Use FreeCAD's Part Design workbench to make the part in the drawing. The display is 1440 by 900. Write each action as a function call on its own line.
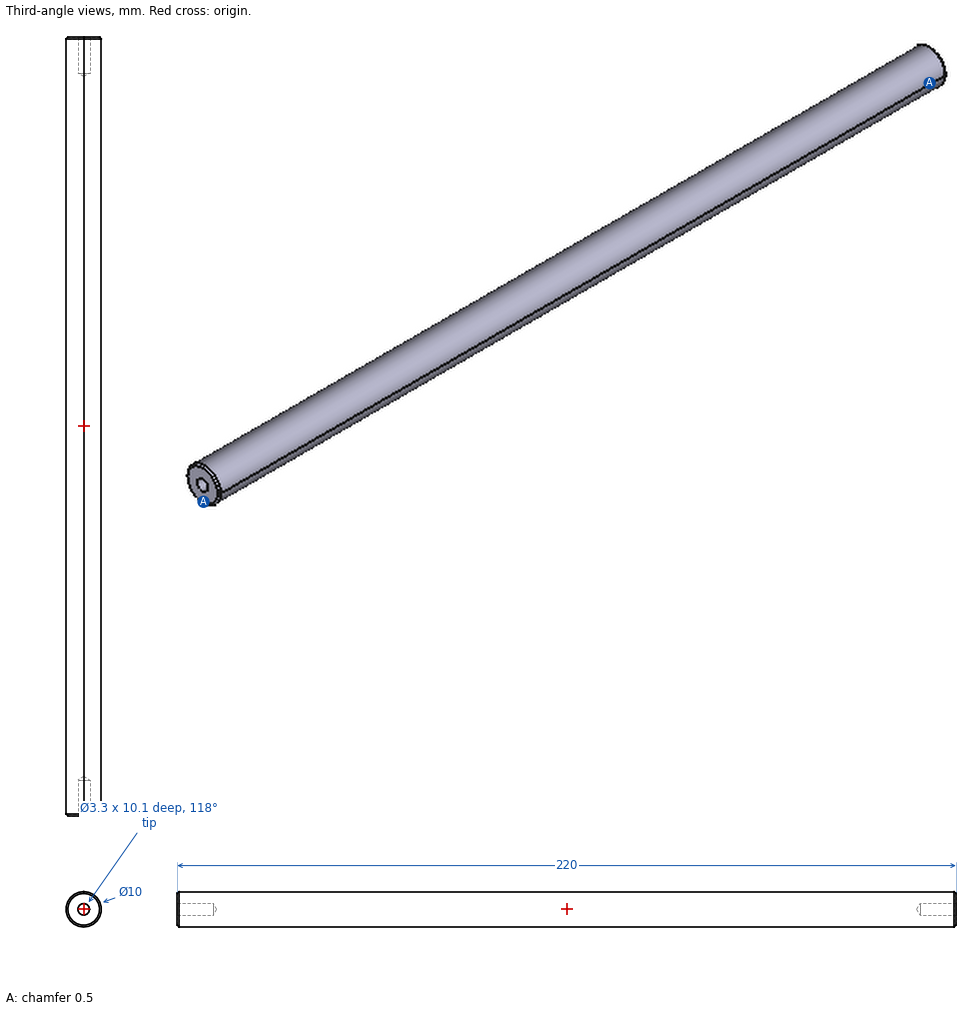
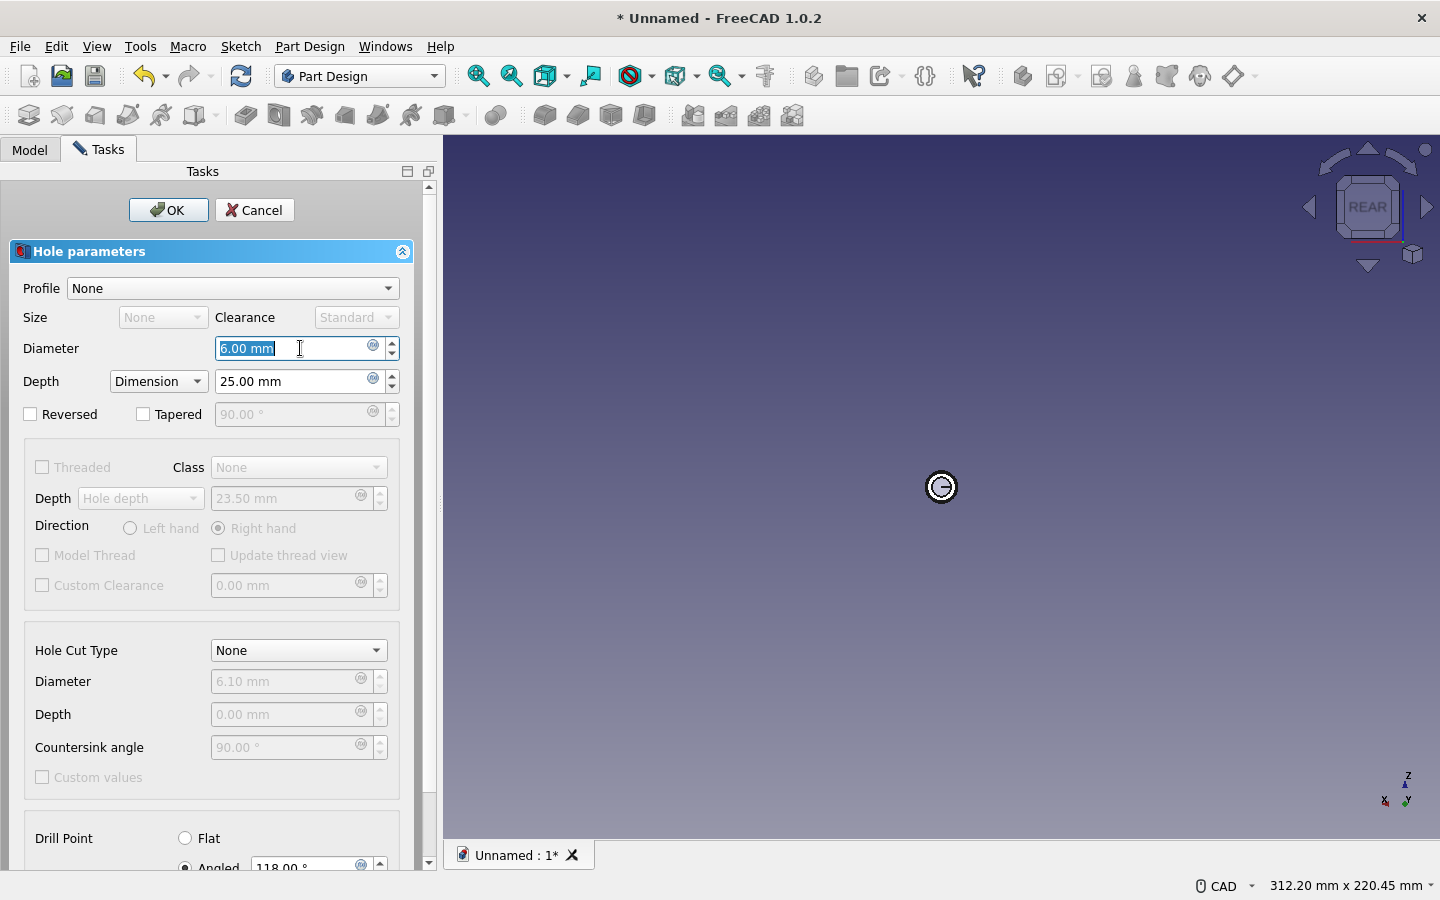
text(3.3)
key(Tab)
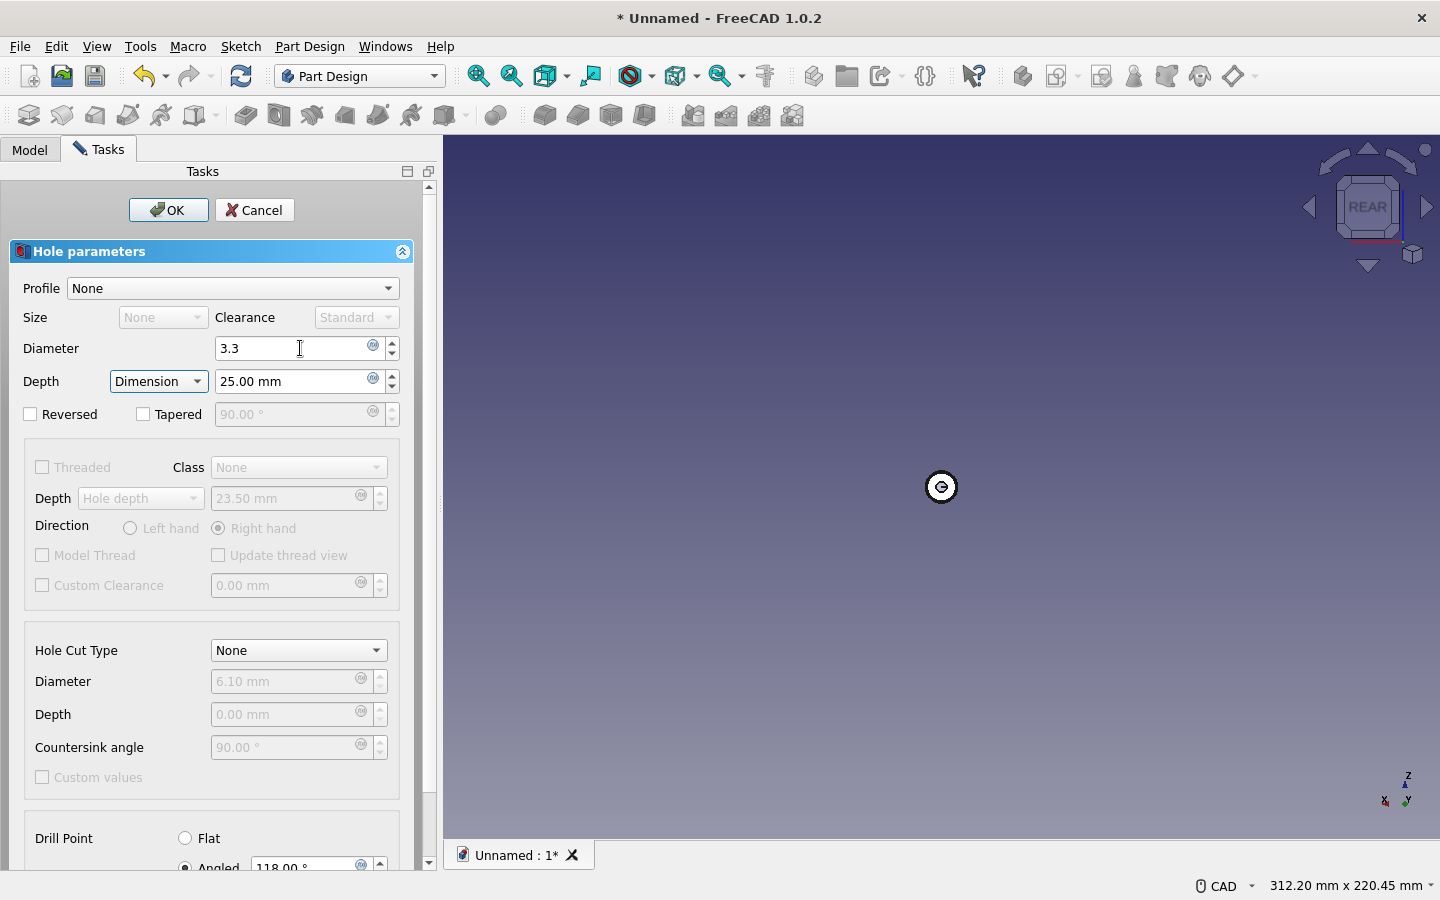
triple_click(300, 382)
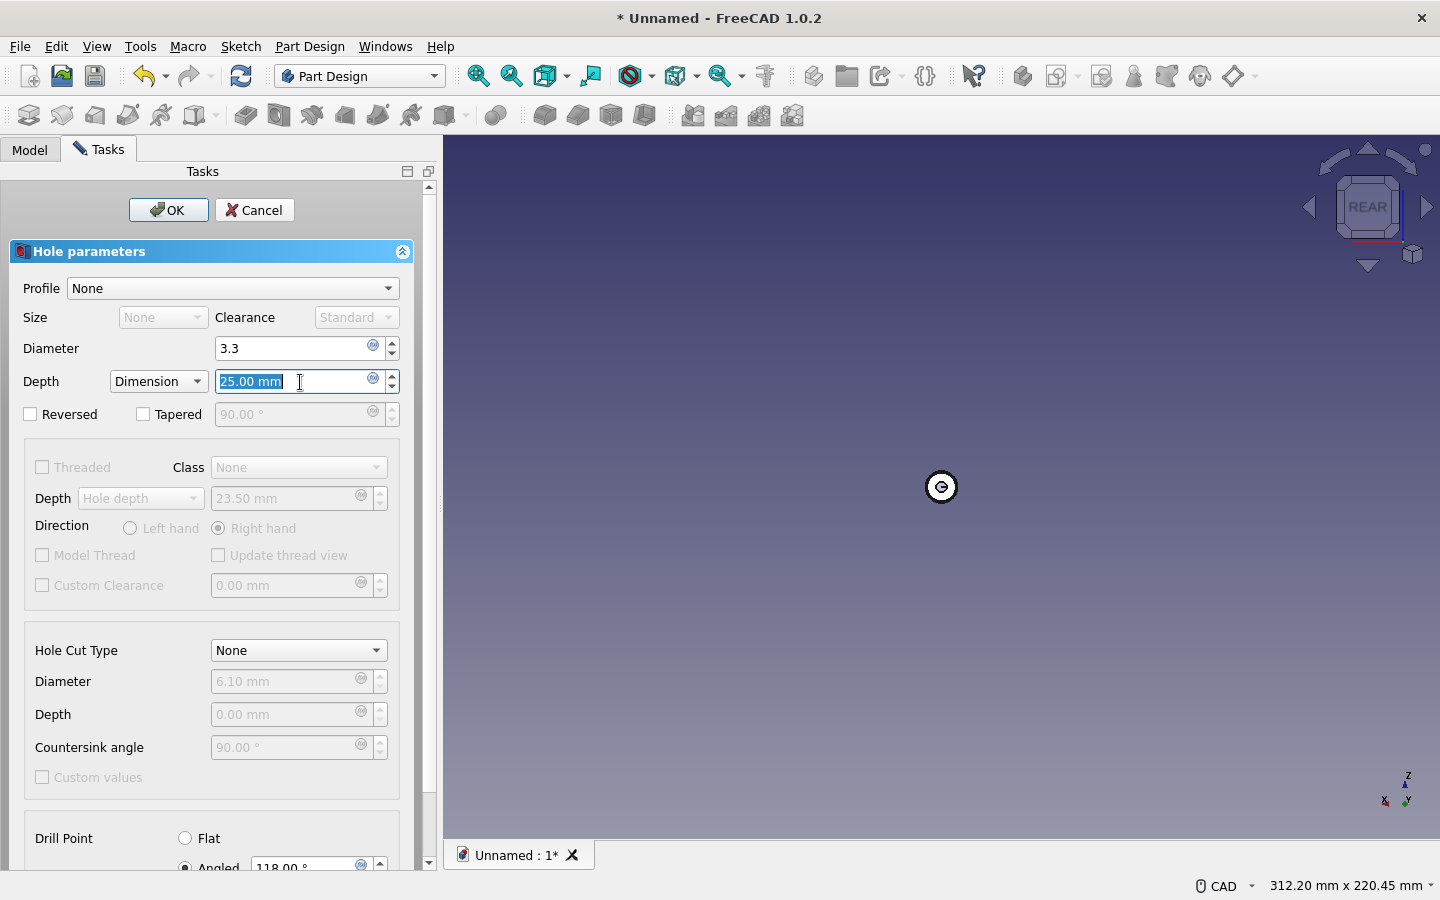
text(10.1)
key(Tab)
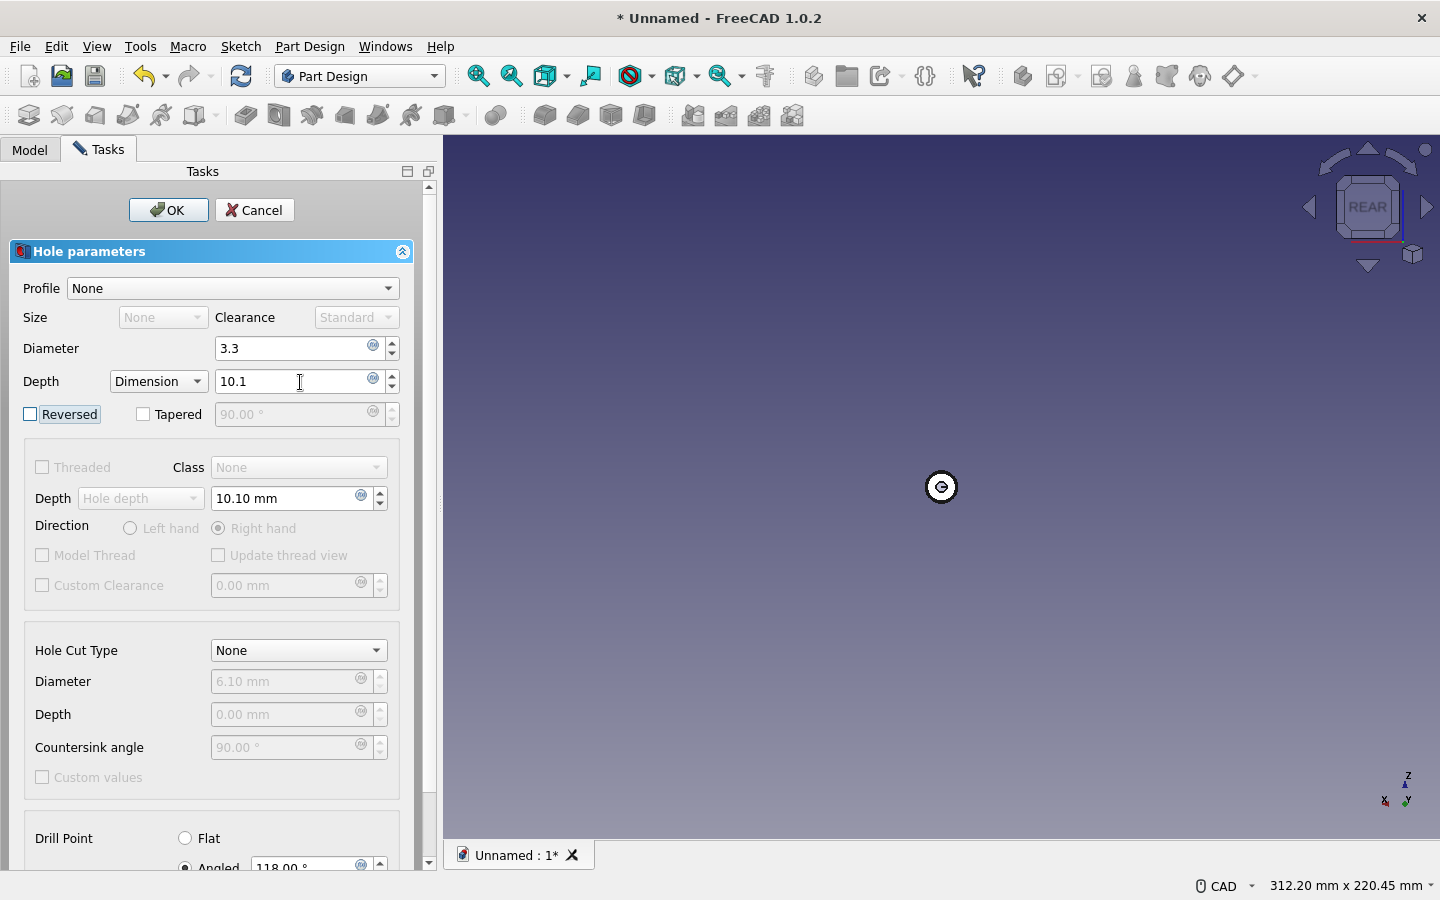
click(169, 210)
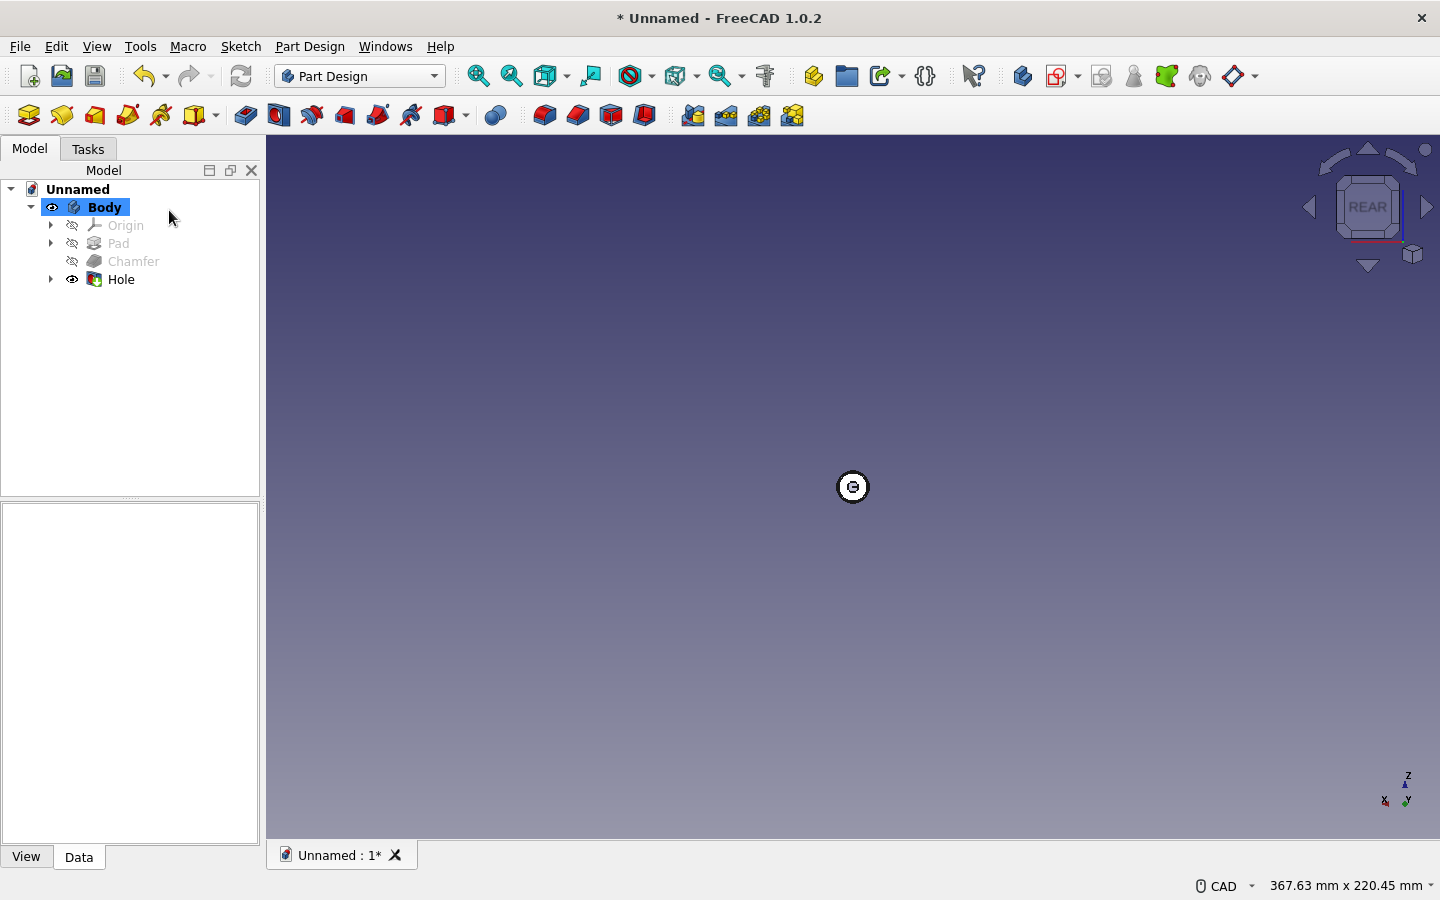
click(479, 76)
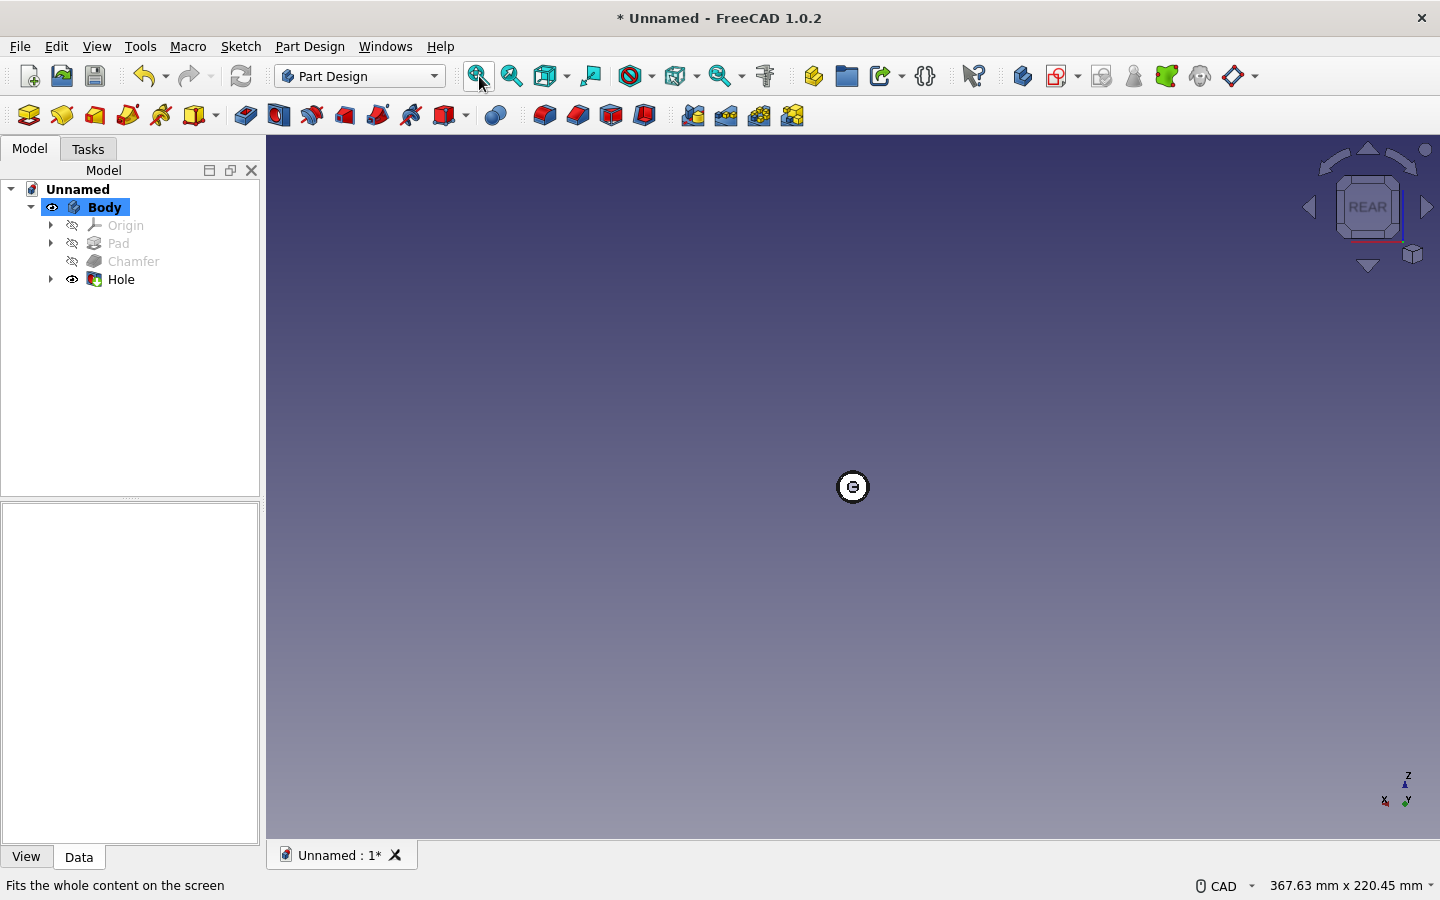
key(0)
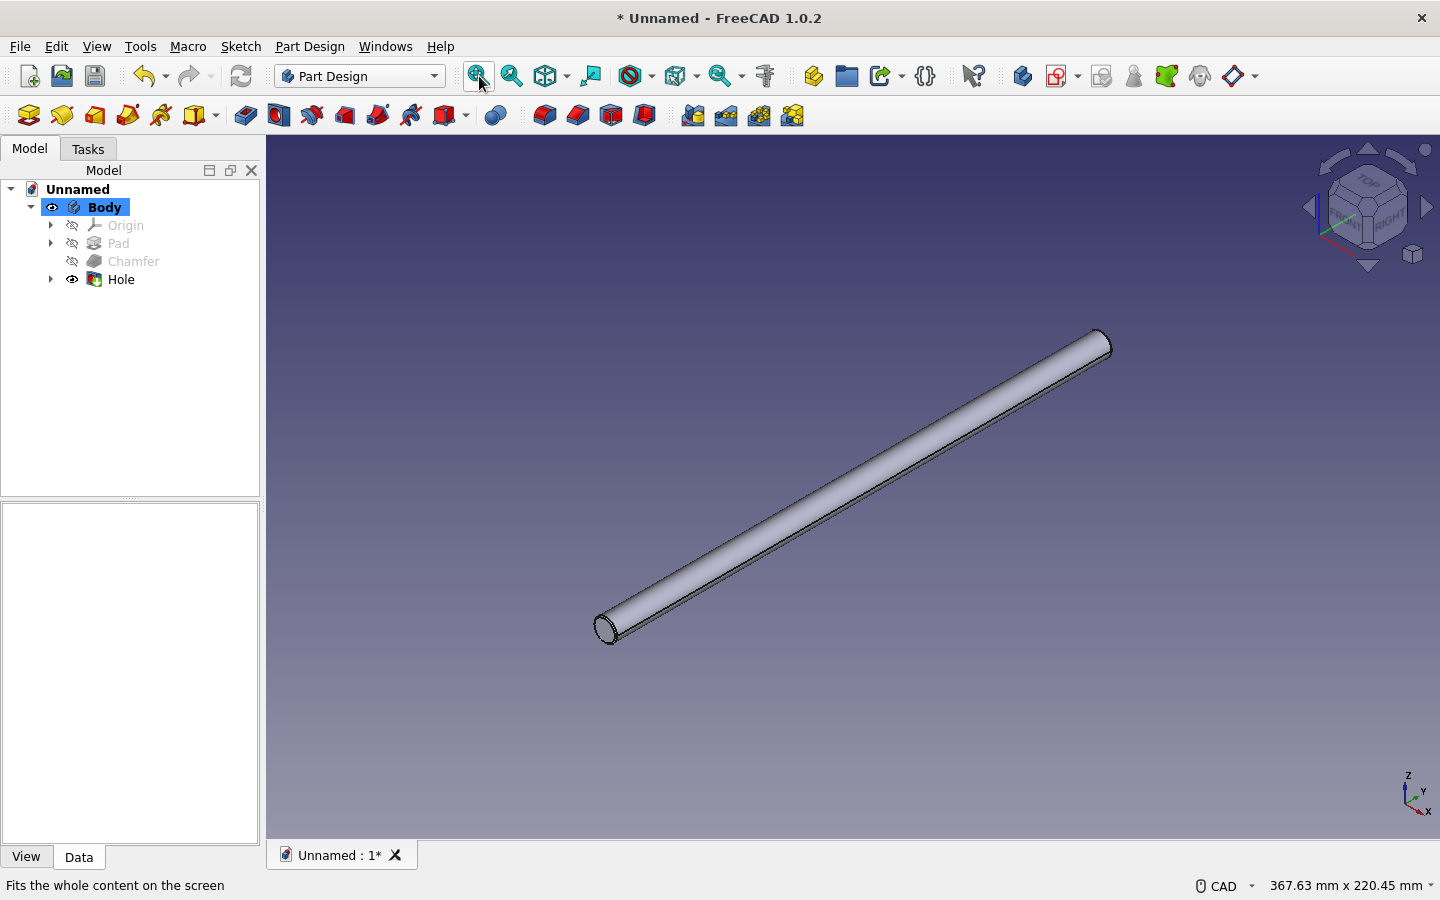
click(605, 633)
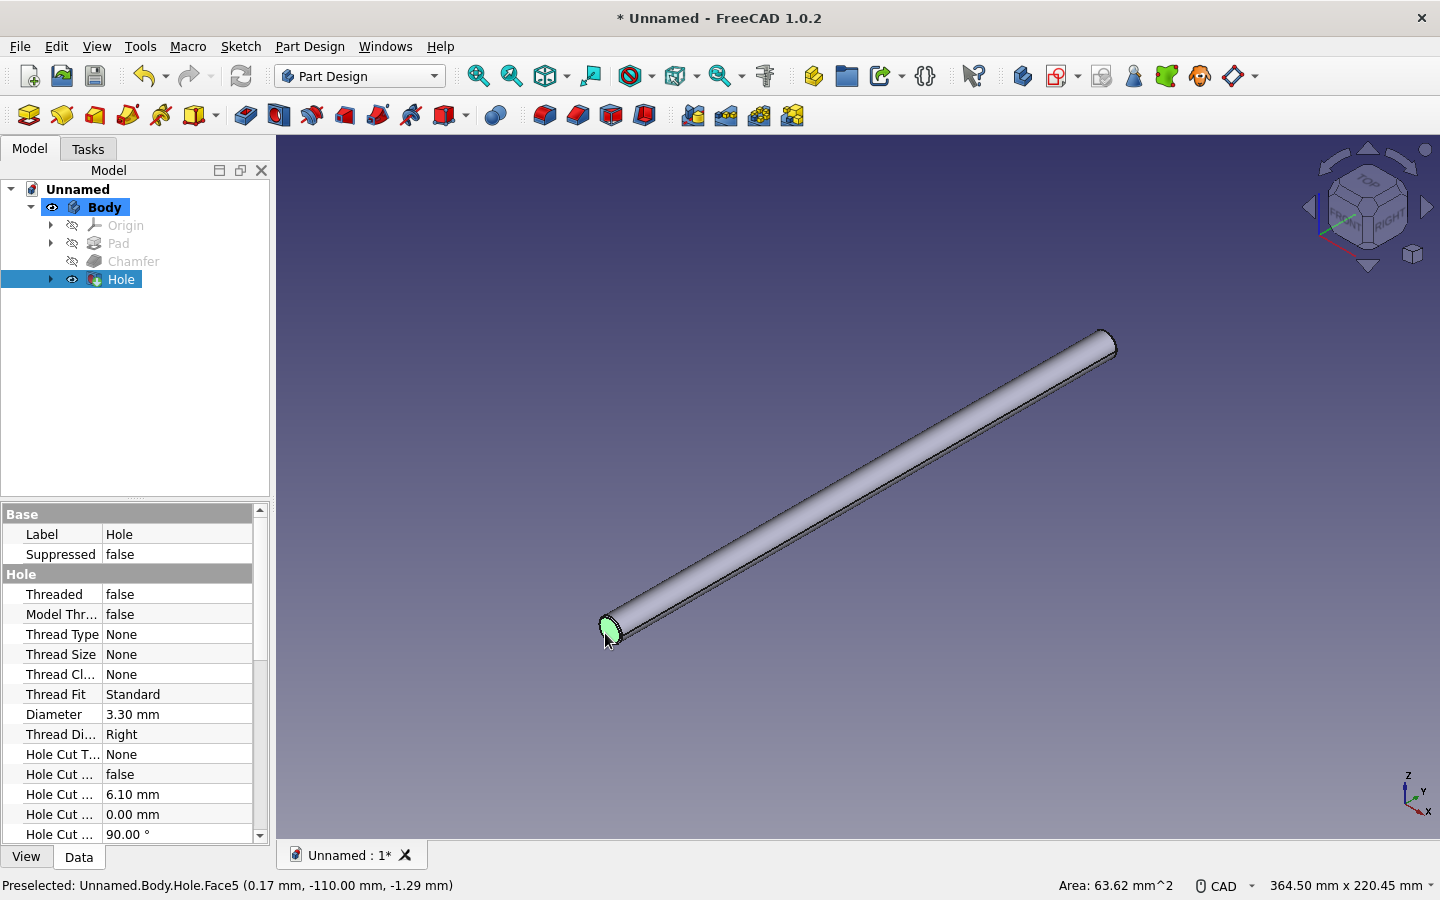
click(1056, 76)